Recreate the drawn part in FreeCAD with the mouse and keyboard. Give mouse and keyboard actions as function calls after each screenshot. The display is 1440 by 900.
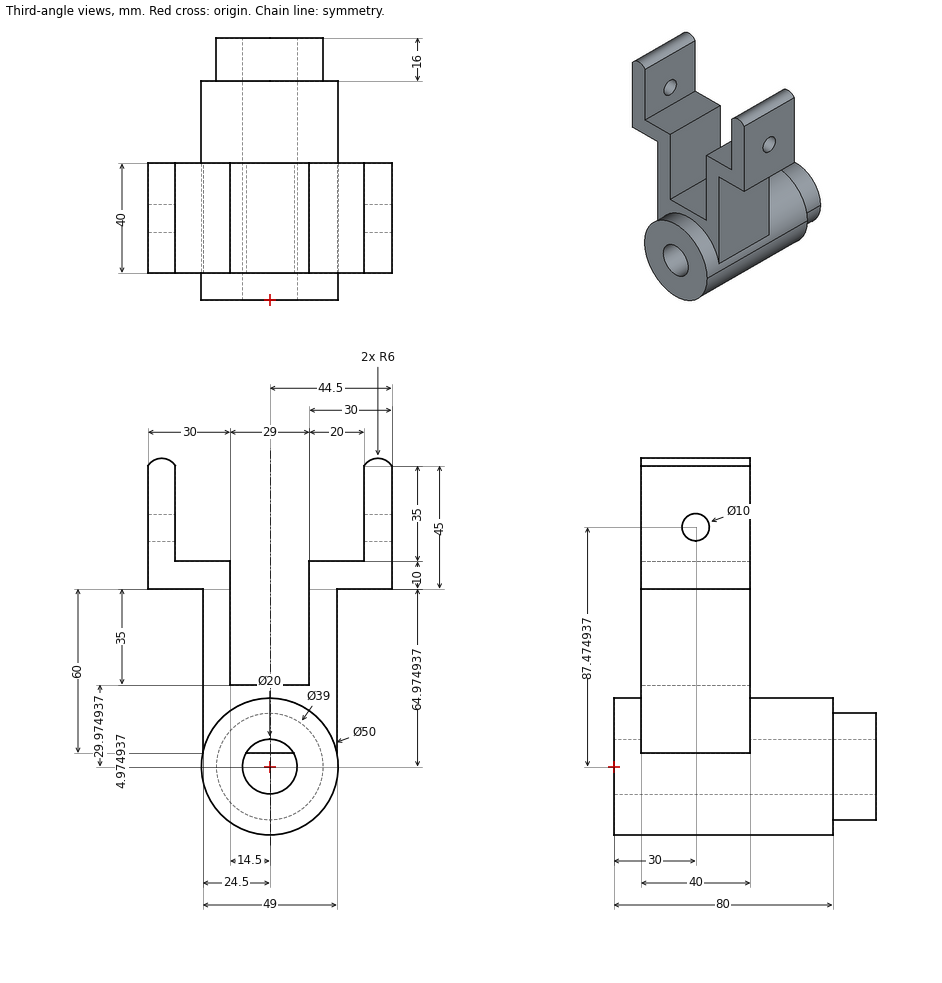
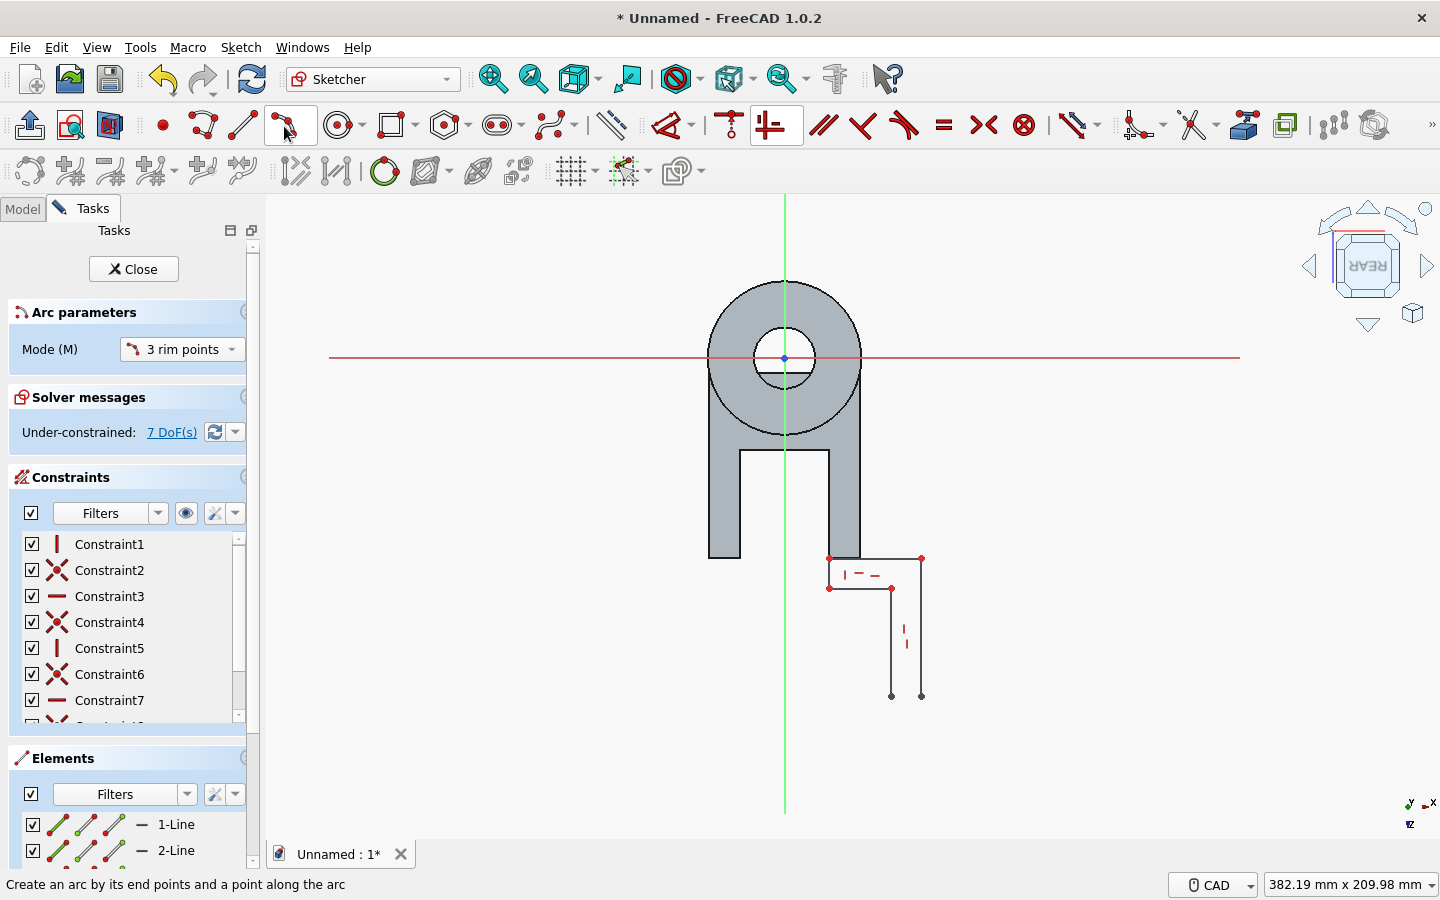
click(891, 697)
click(921, 697)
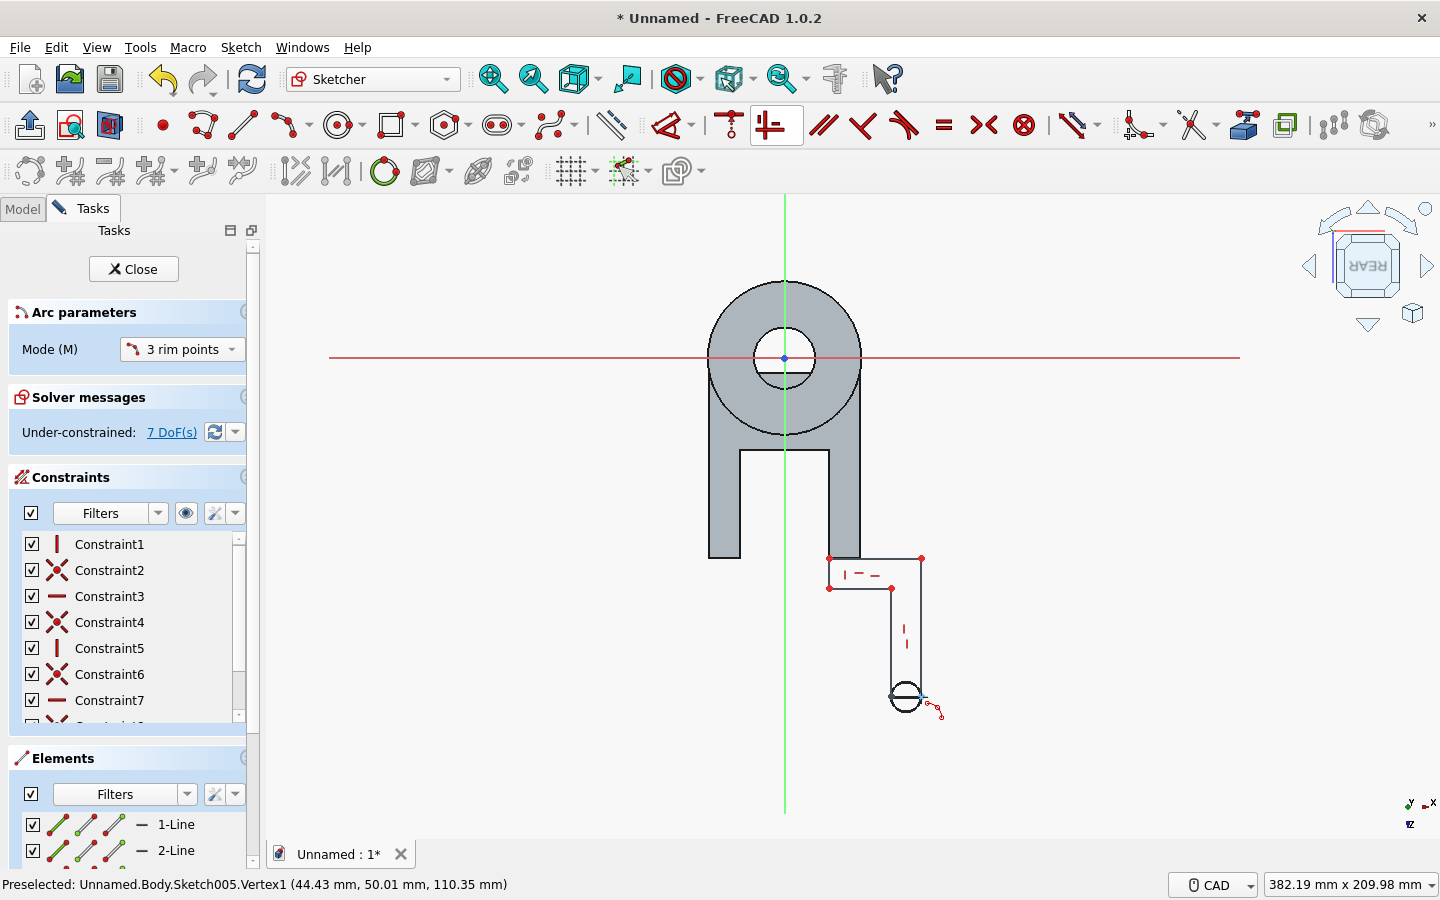
scroll(906, 704, up, 4)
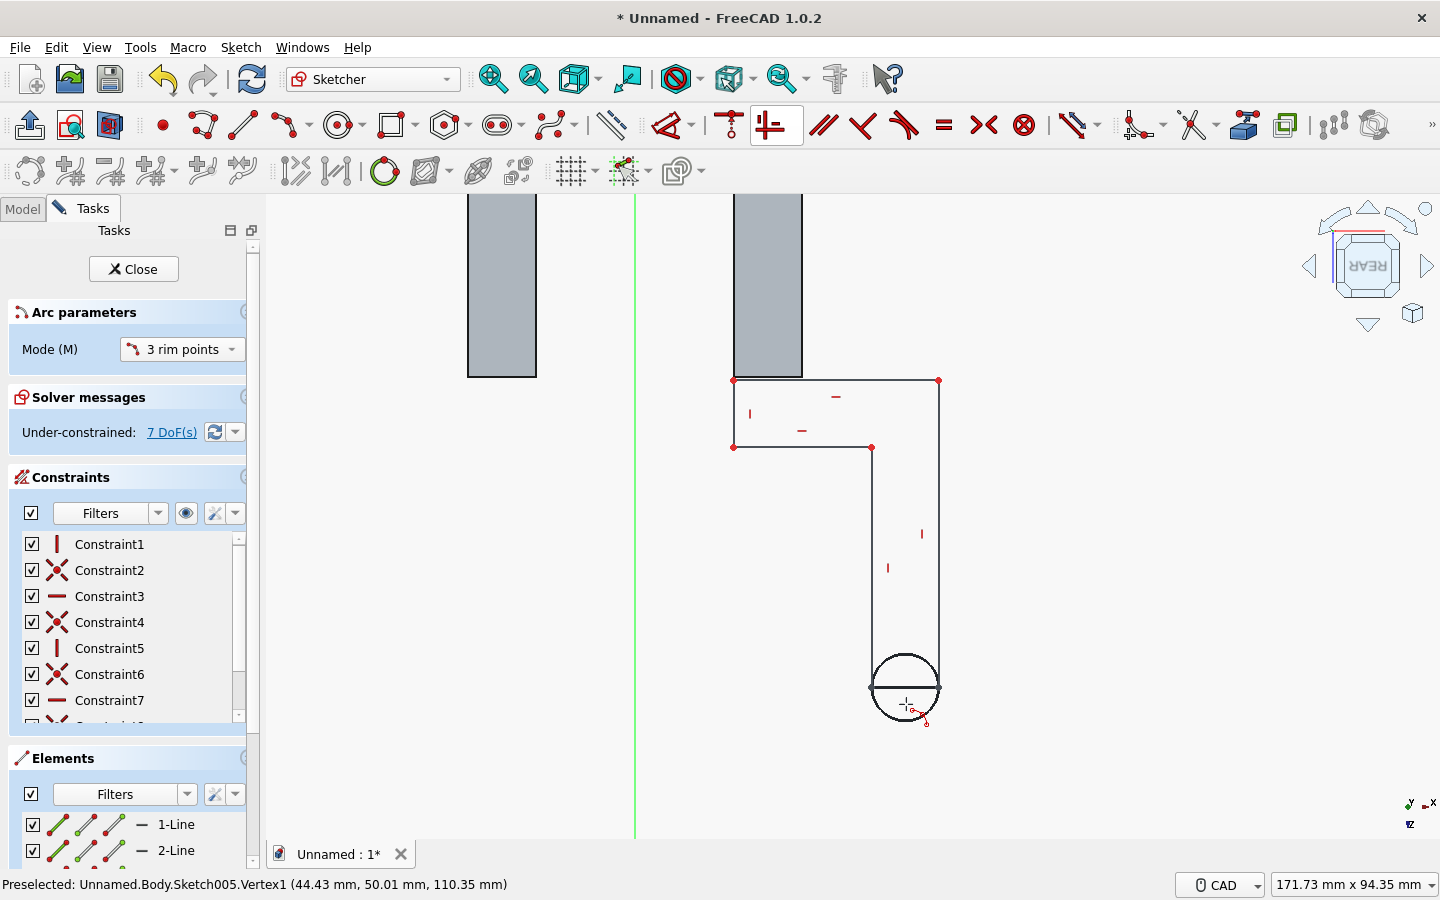
click(905, 703)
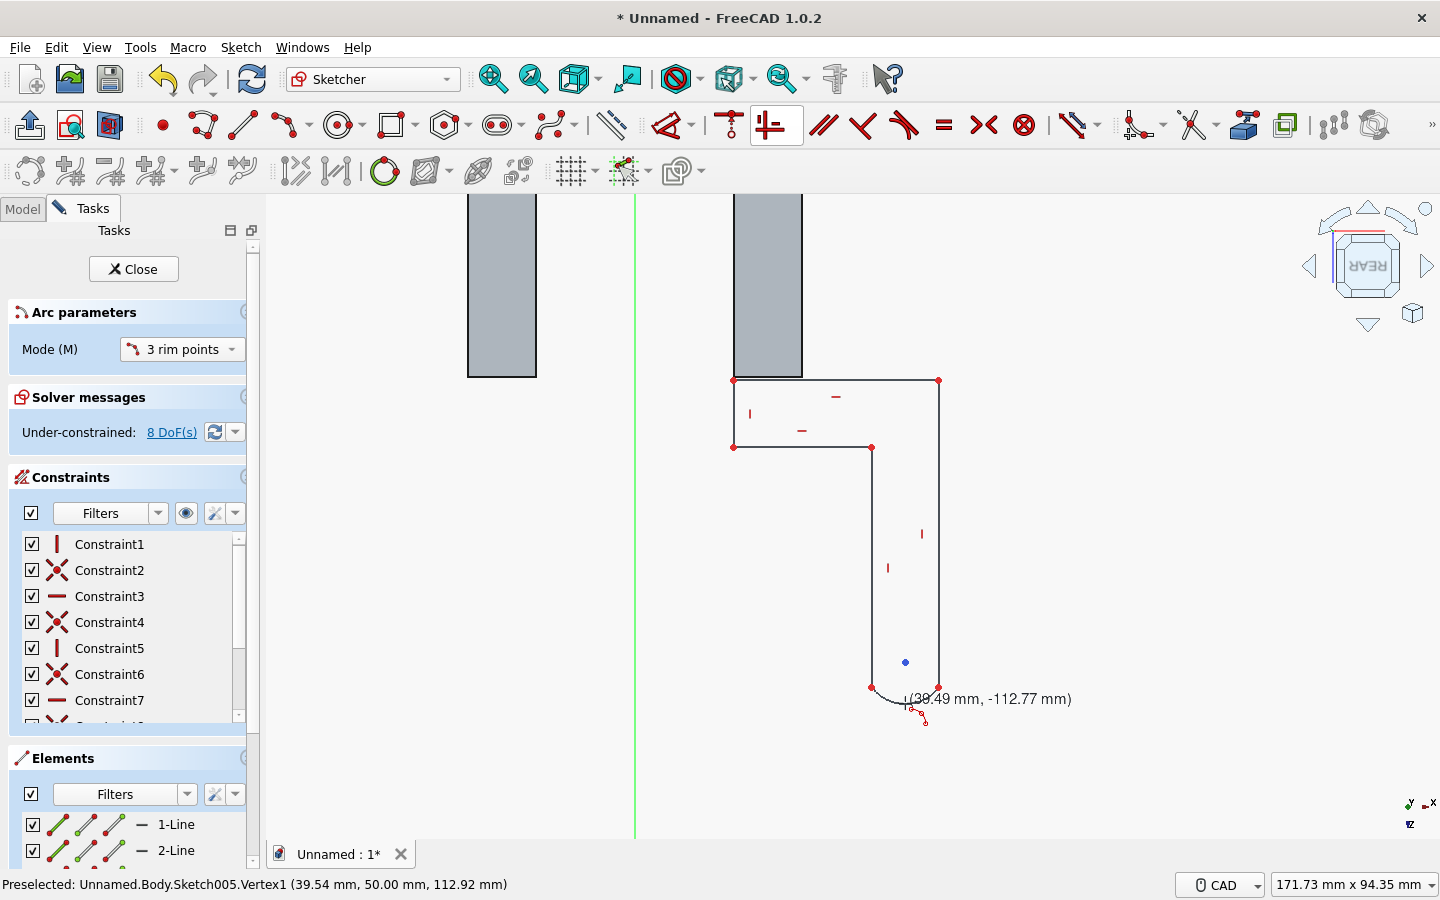
click(204, 126)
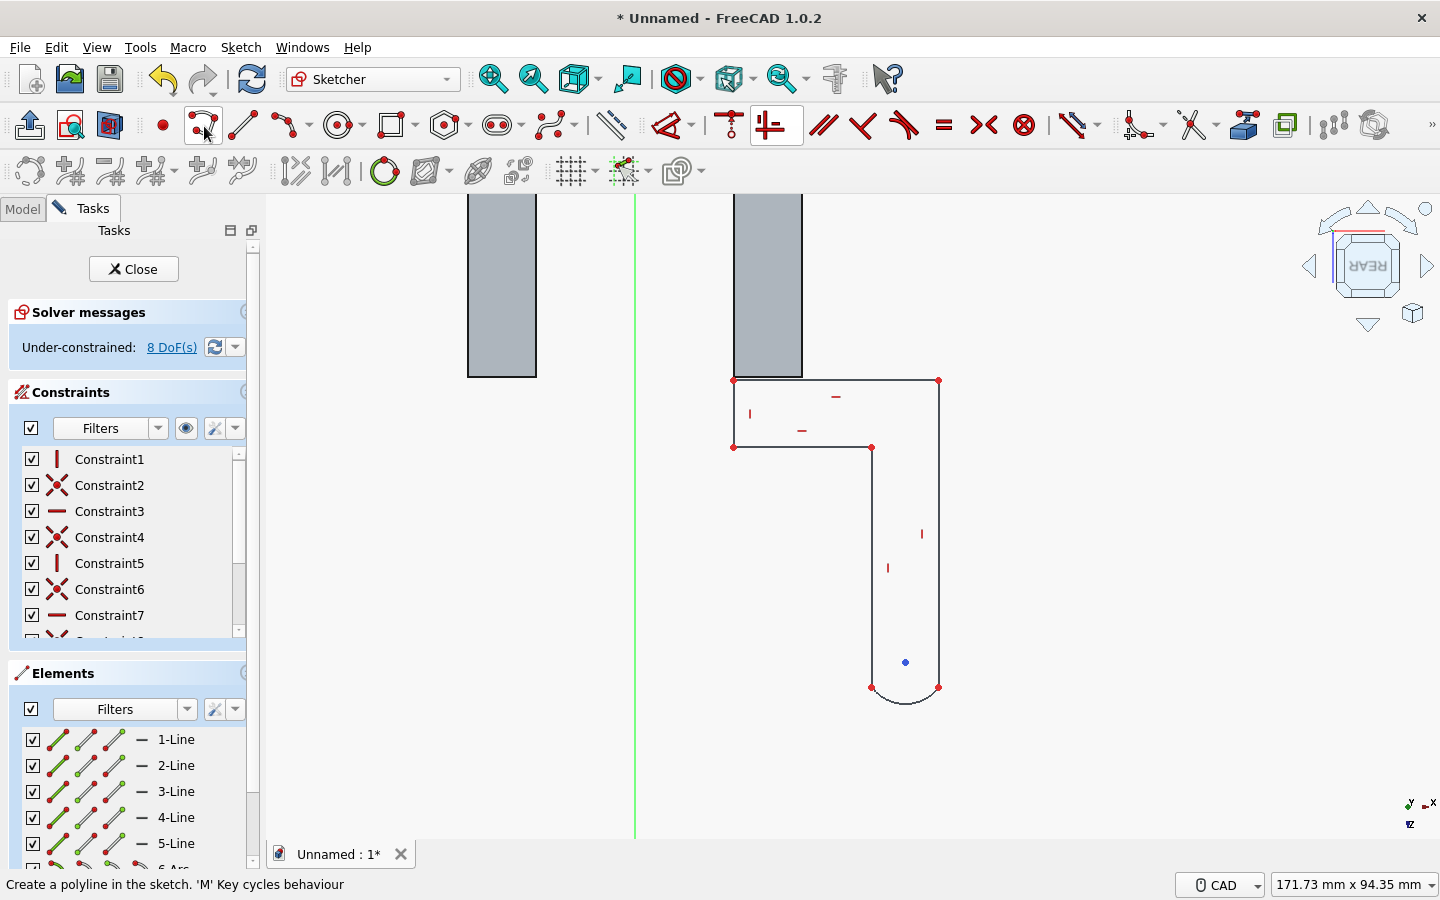
click(399, 685)
click(399, 446)
click(536, 446)
click(536, 377)
click(331, 377)
click(331, 685)
right_click(331, 685)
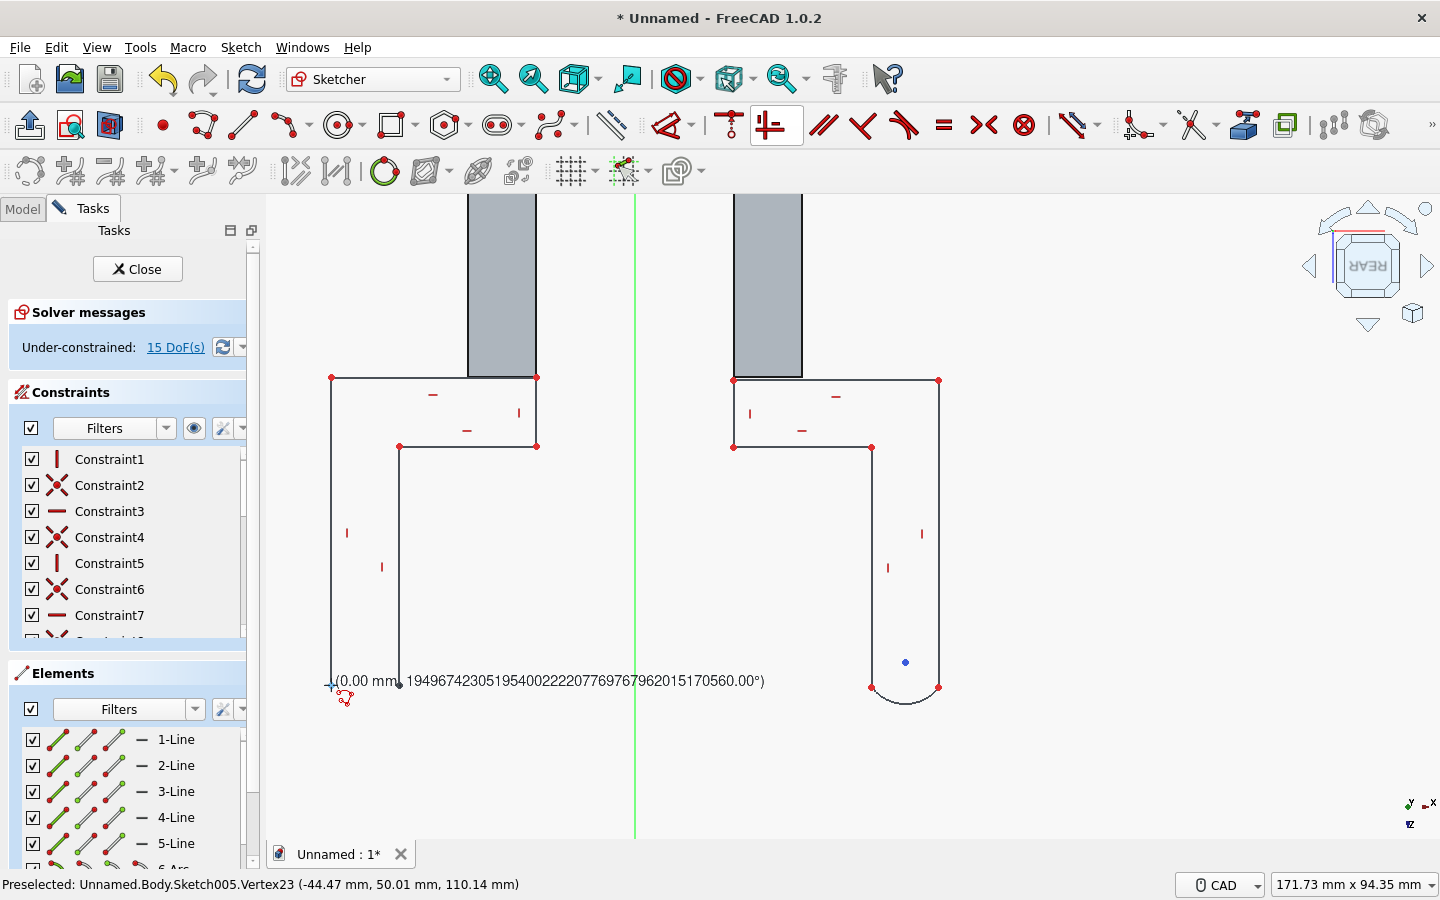
click(284, 126)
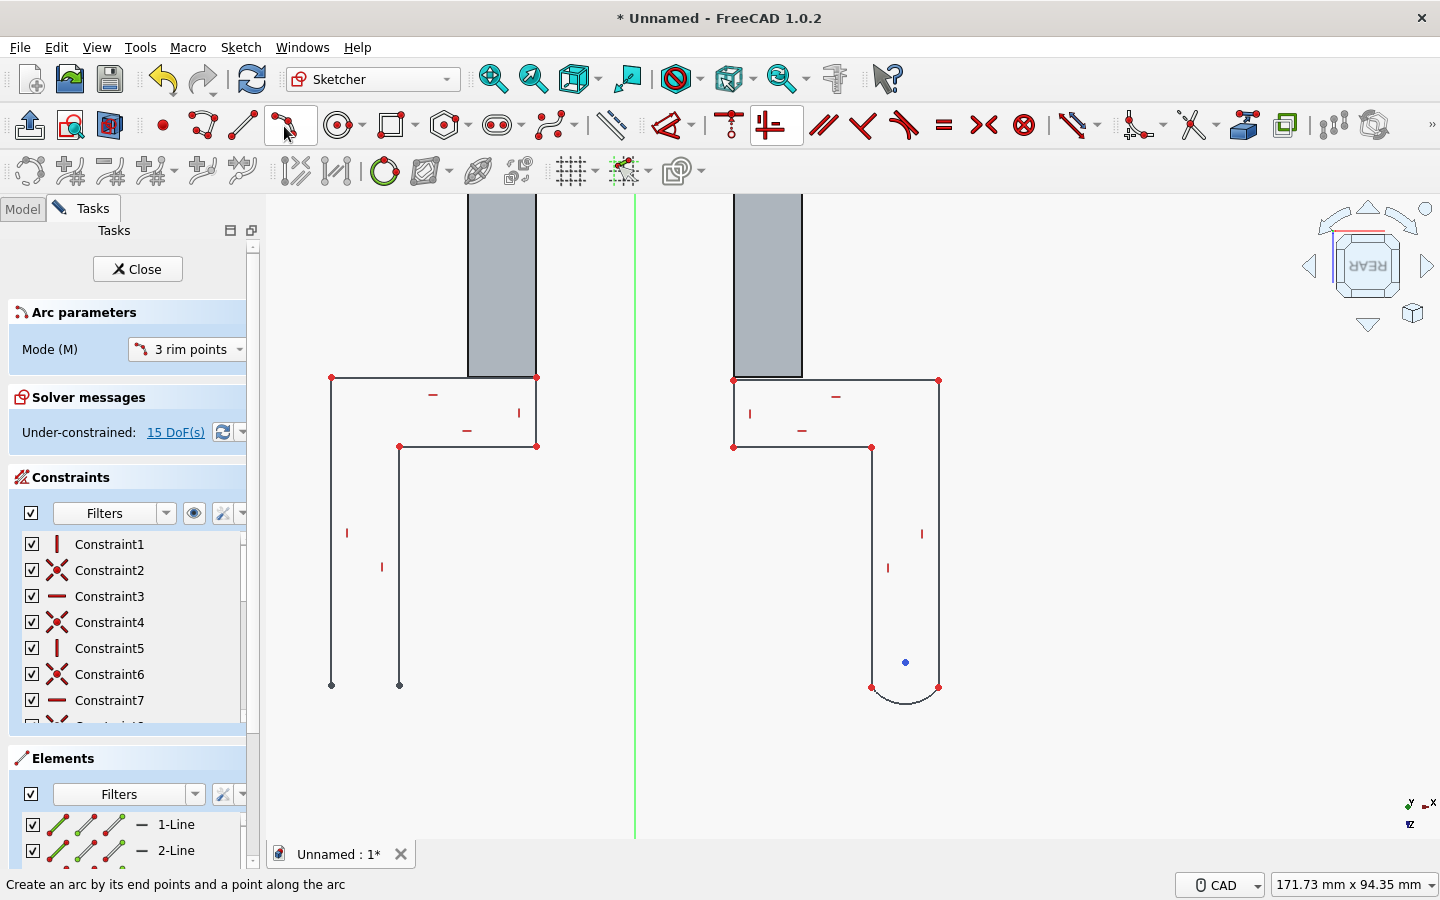
click(331, 686)
click(399, 686)
click(365, 703)
key(Escape)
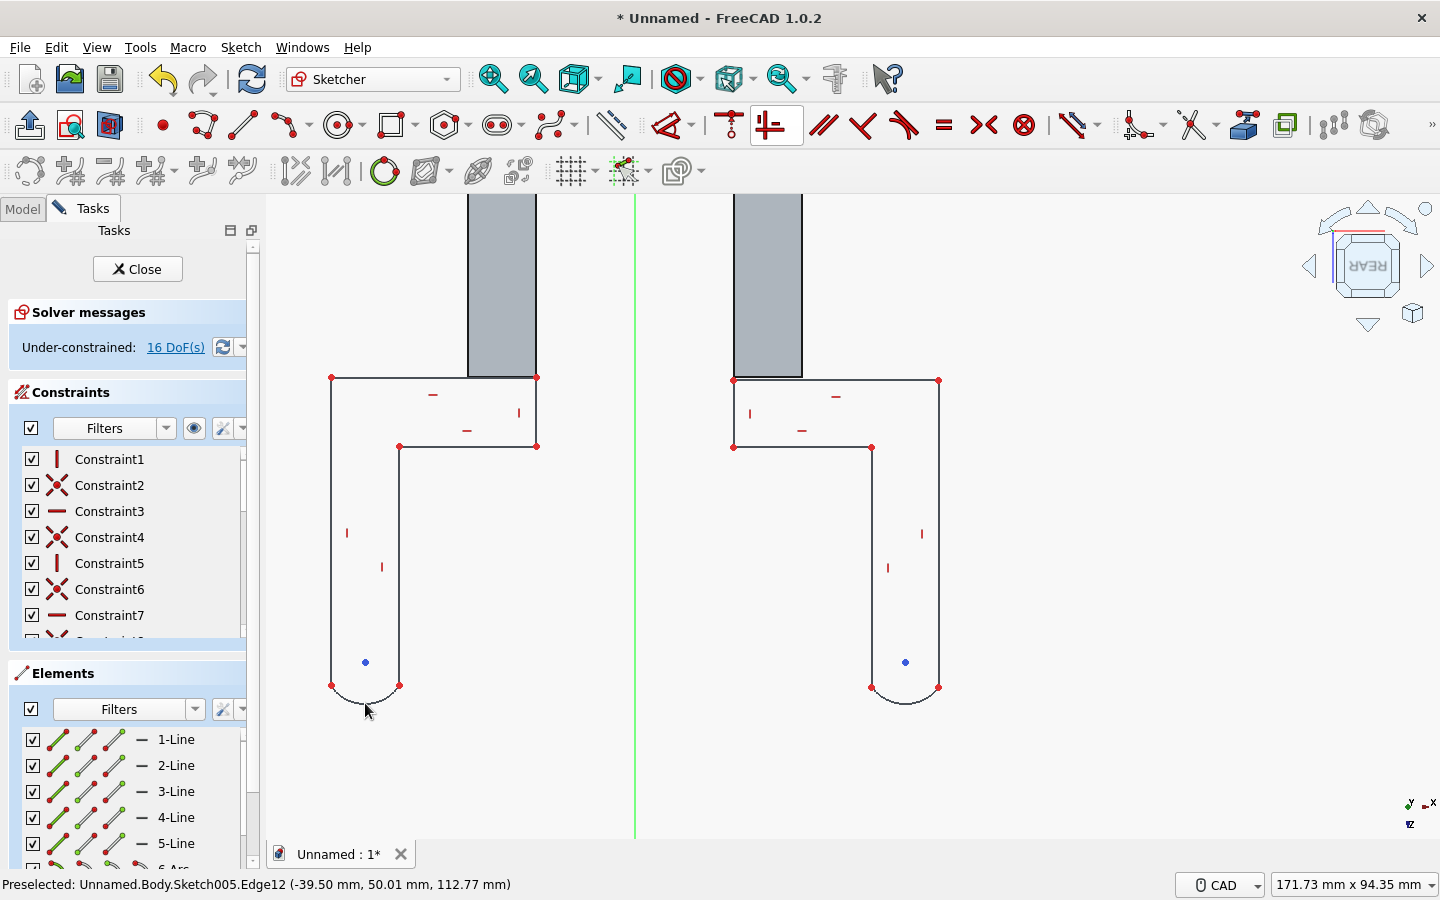
click(890, 701)